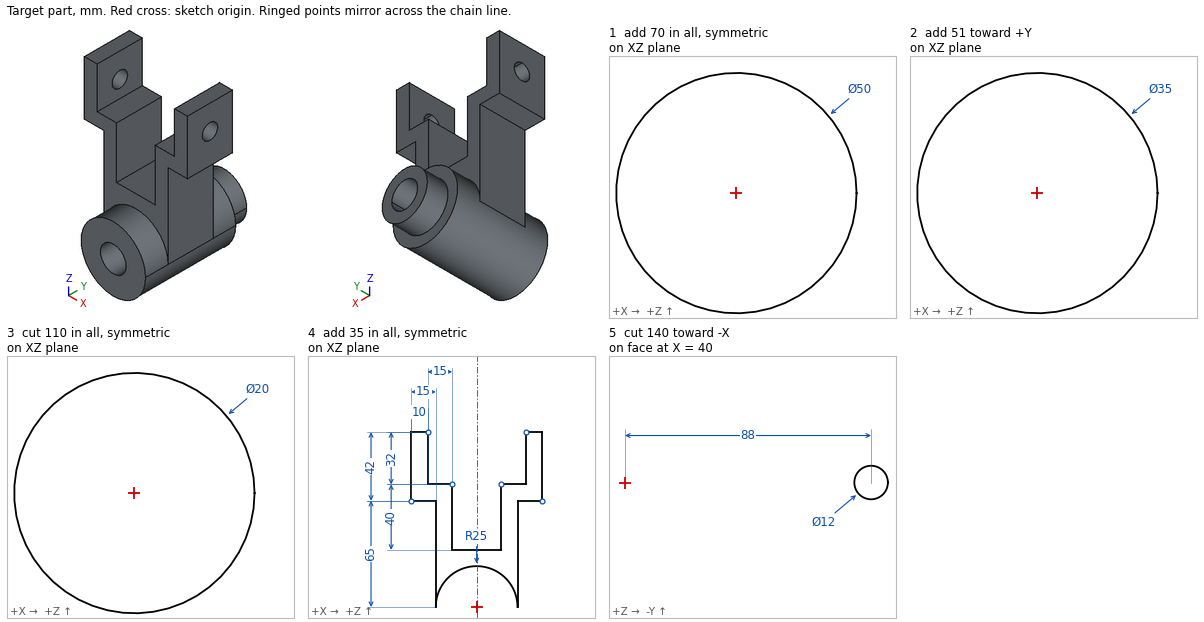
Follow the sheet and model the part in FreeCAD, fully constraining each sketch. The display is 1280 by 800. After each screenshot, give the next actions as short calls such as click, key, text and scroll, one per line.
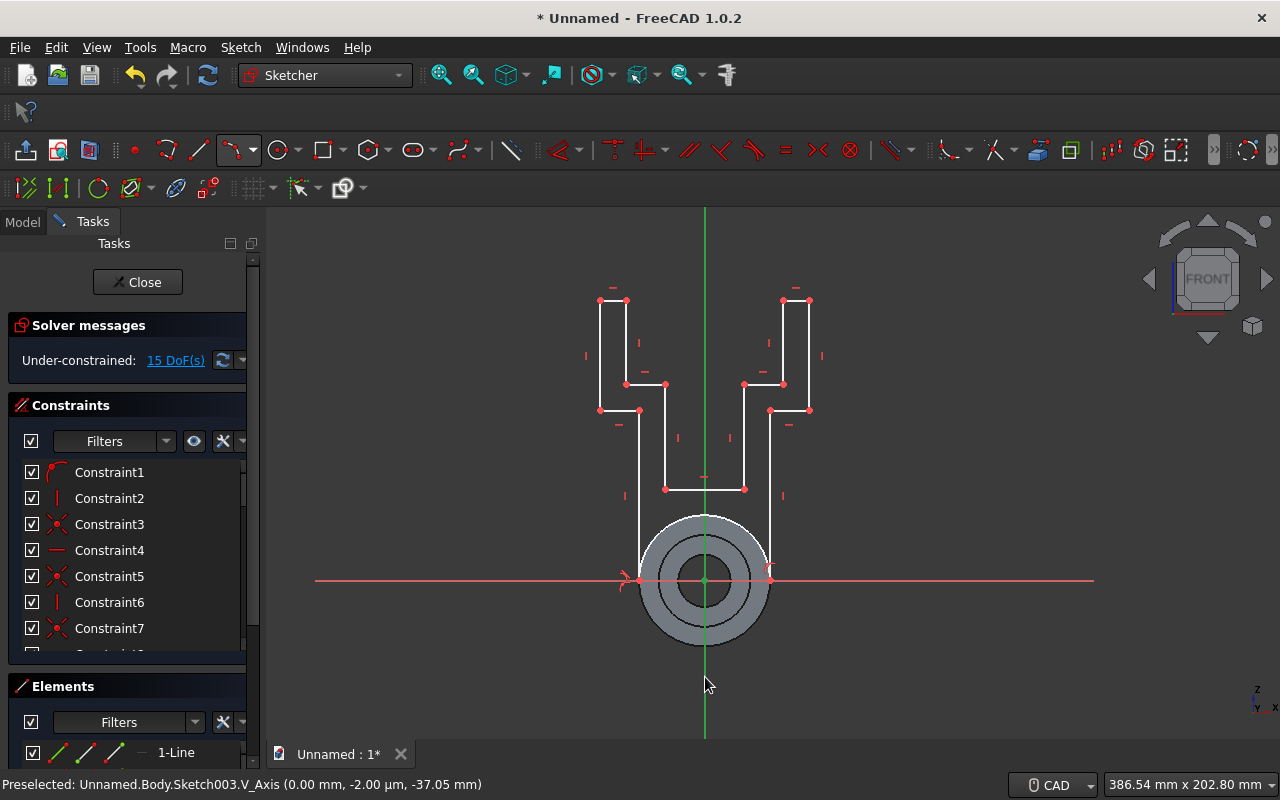
click(614, 150)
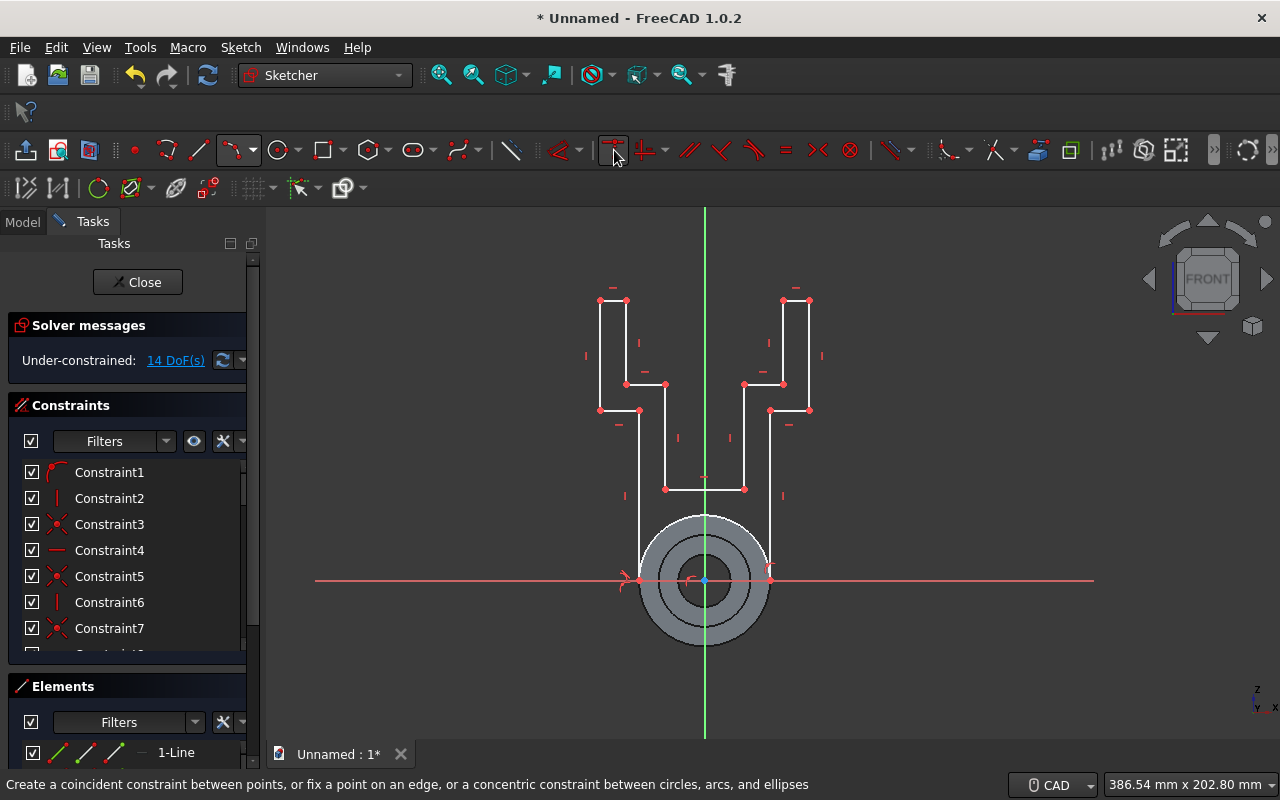
click(665, 385)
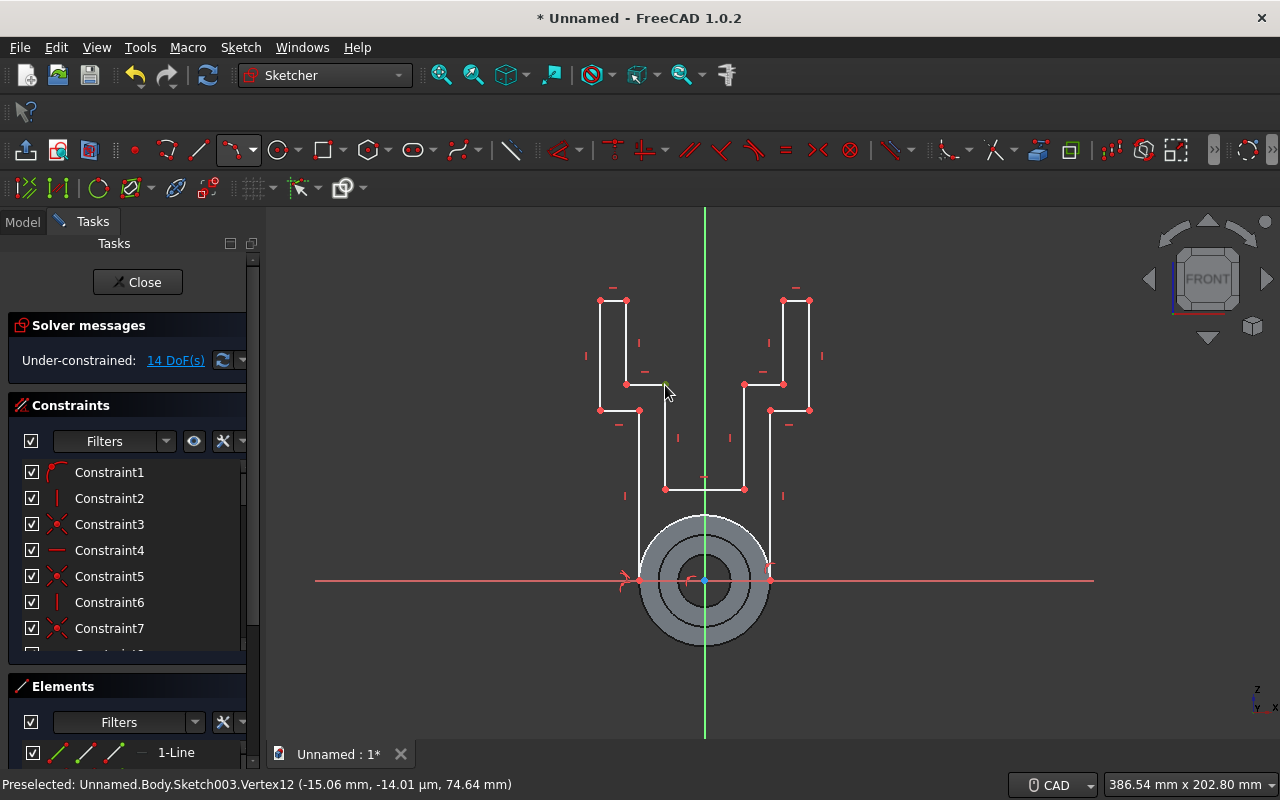
click(744, 385)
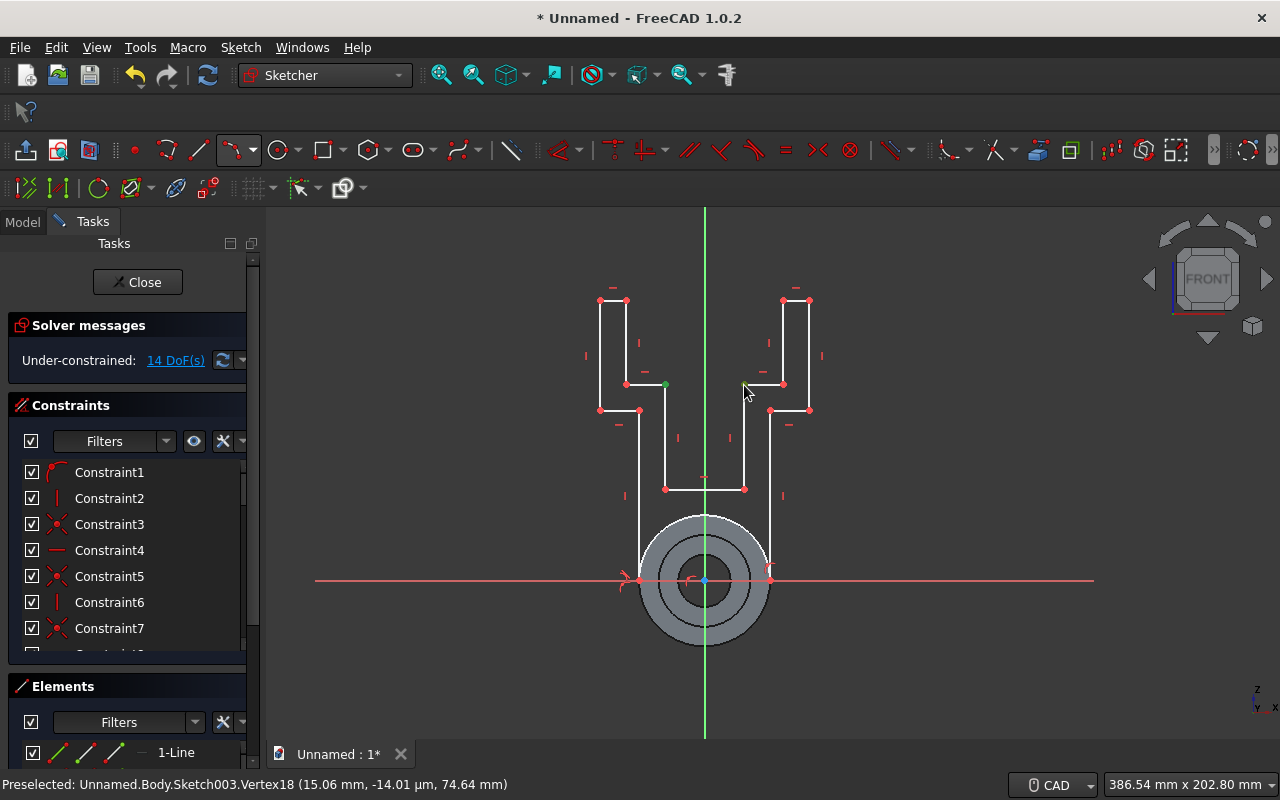
click(705, 677)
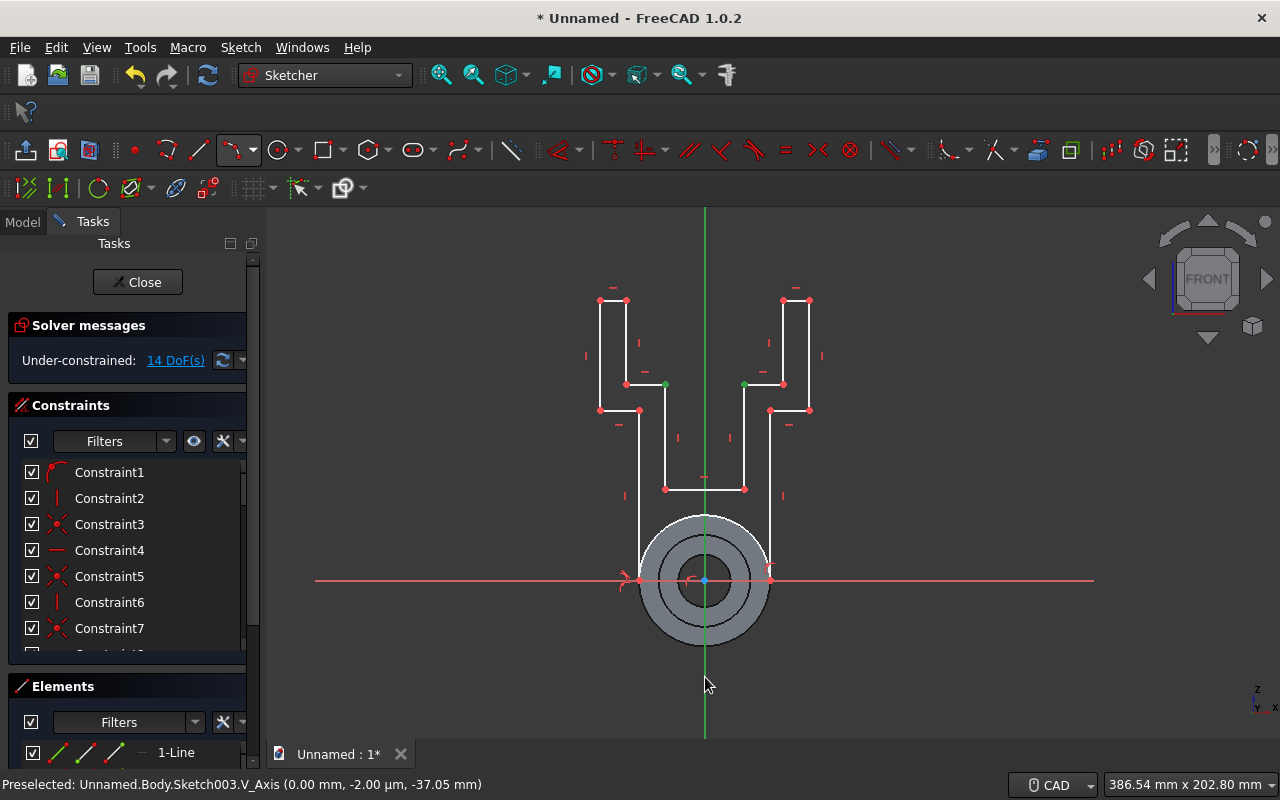
click(818, 150)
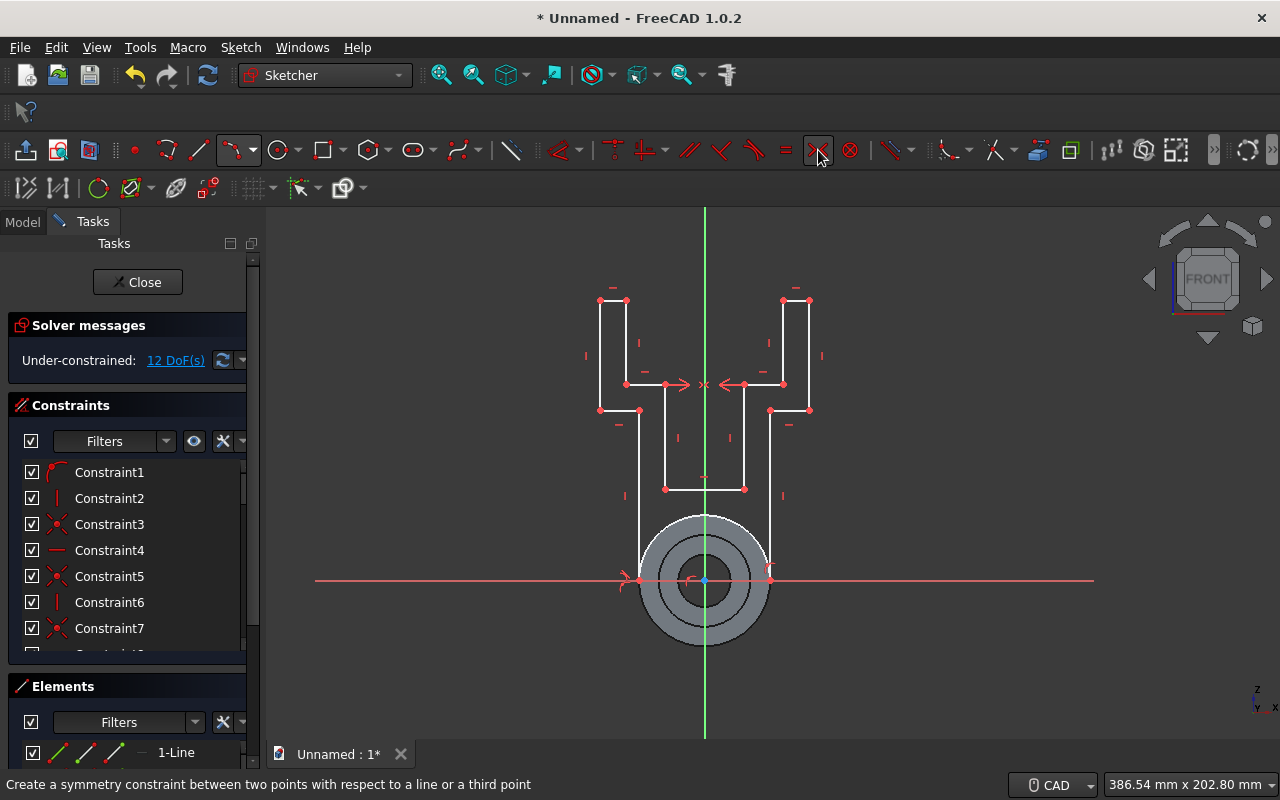
click(626, 301)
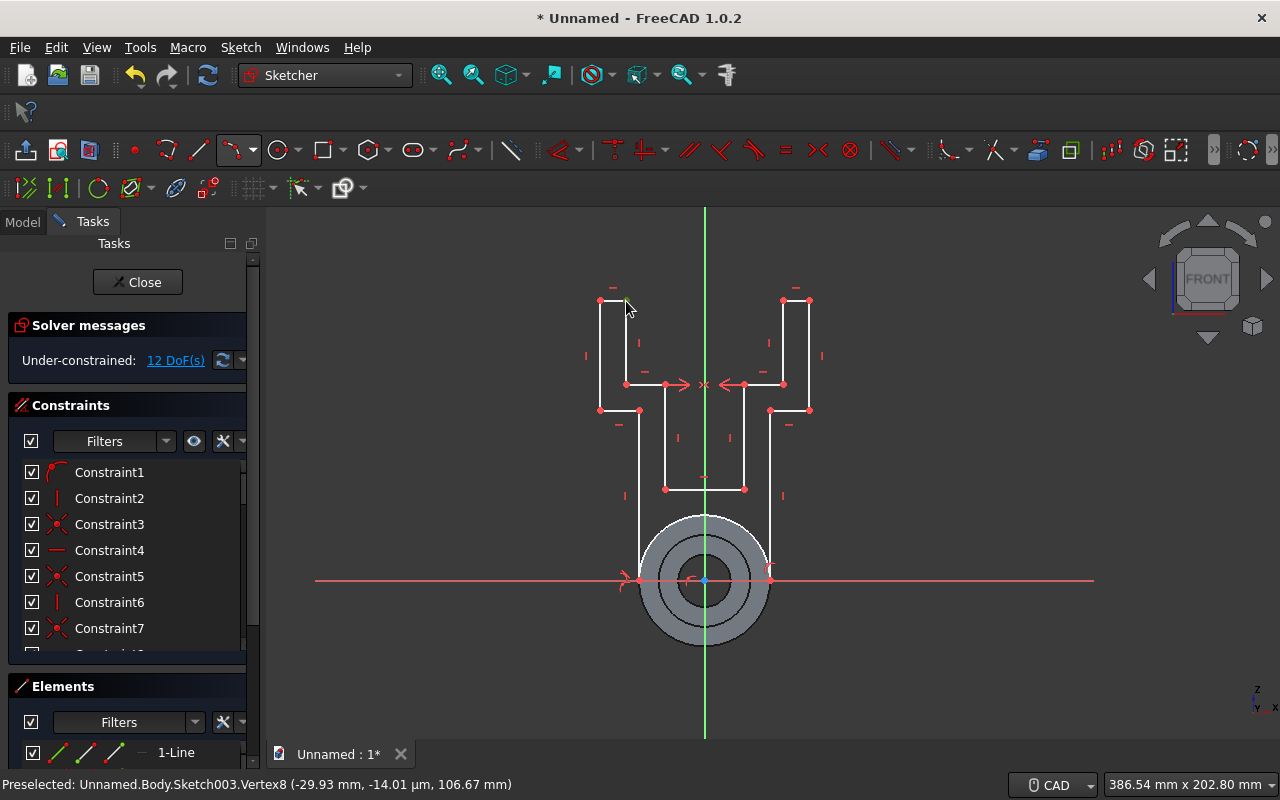
click(783, 301)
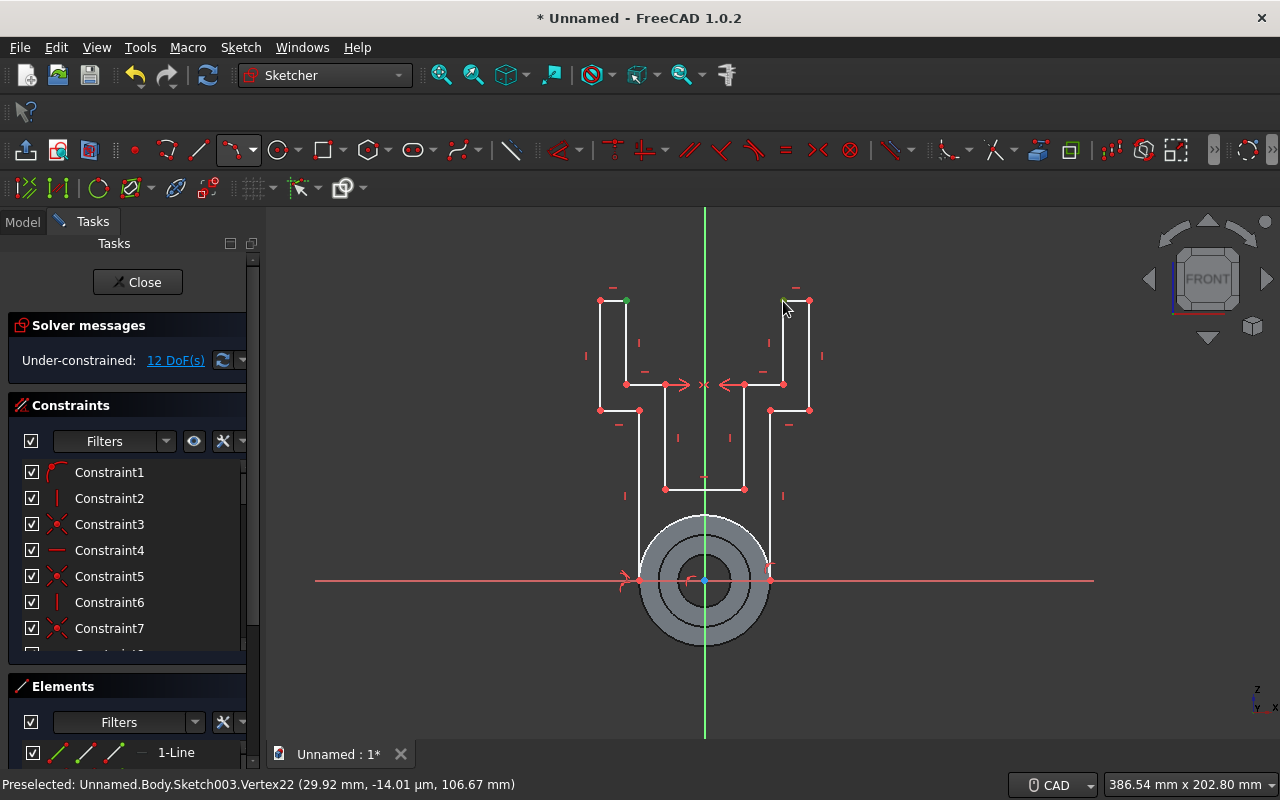
click(705, 677)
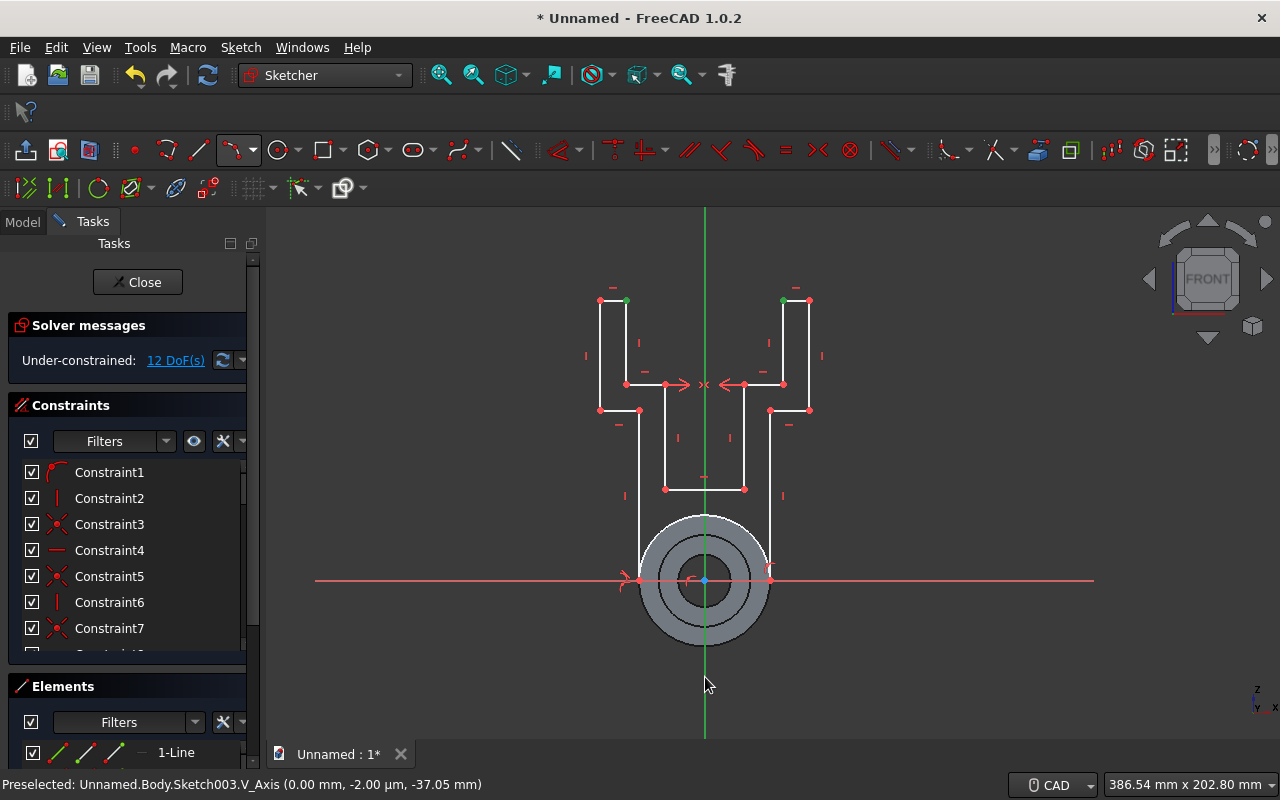
key(s)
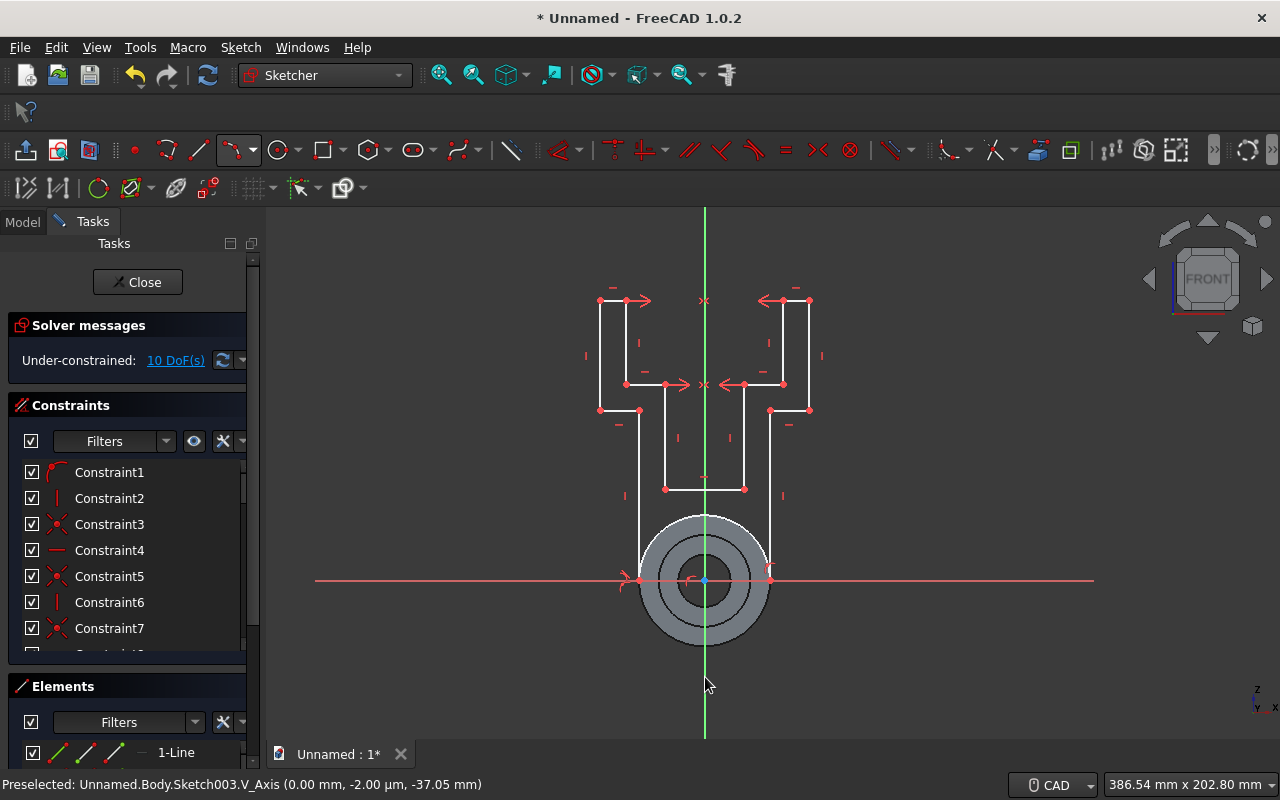
click(600, 411)